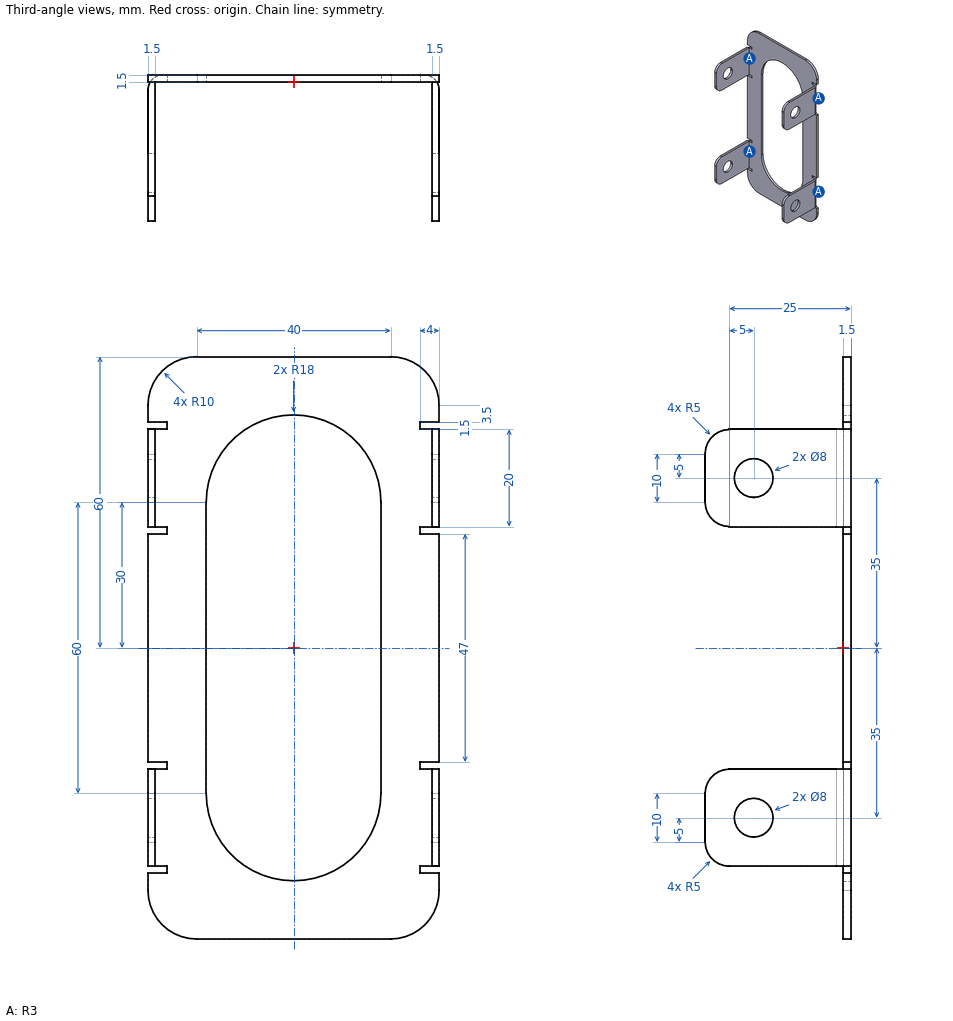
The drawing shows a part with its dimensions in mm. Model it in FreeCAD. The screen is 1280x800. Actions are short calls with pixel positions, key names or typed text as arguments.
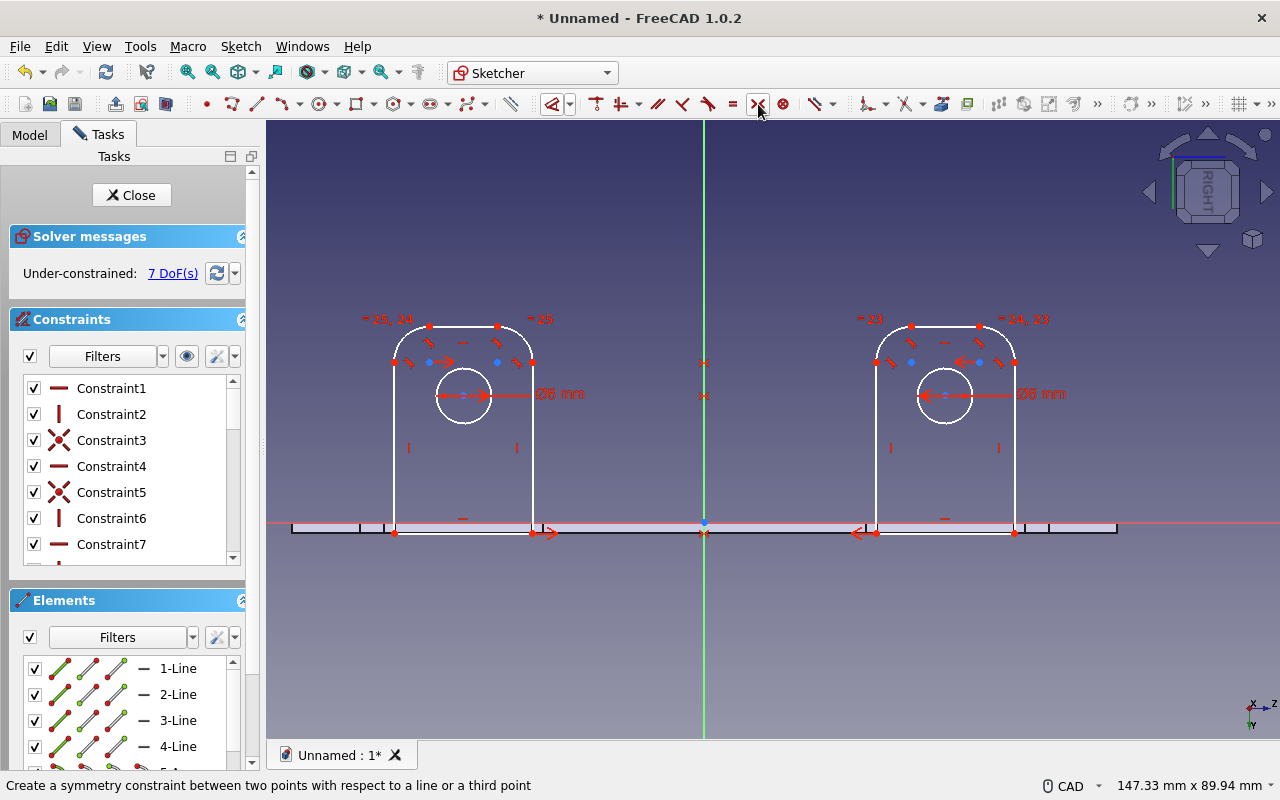
click(896, 331)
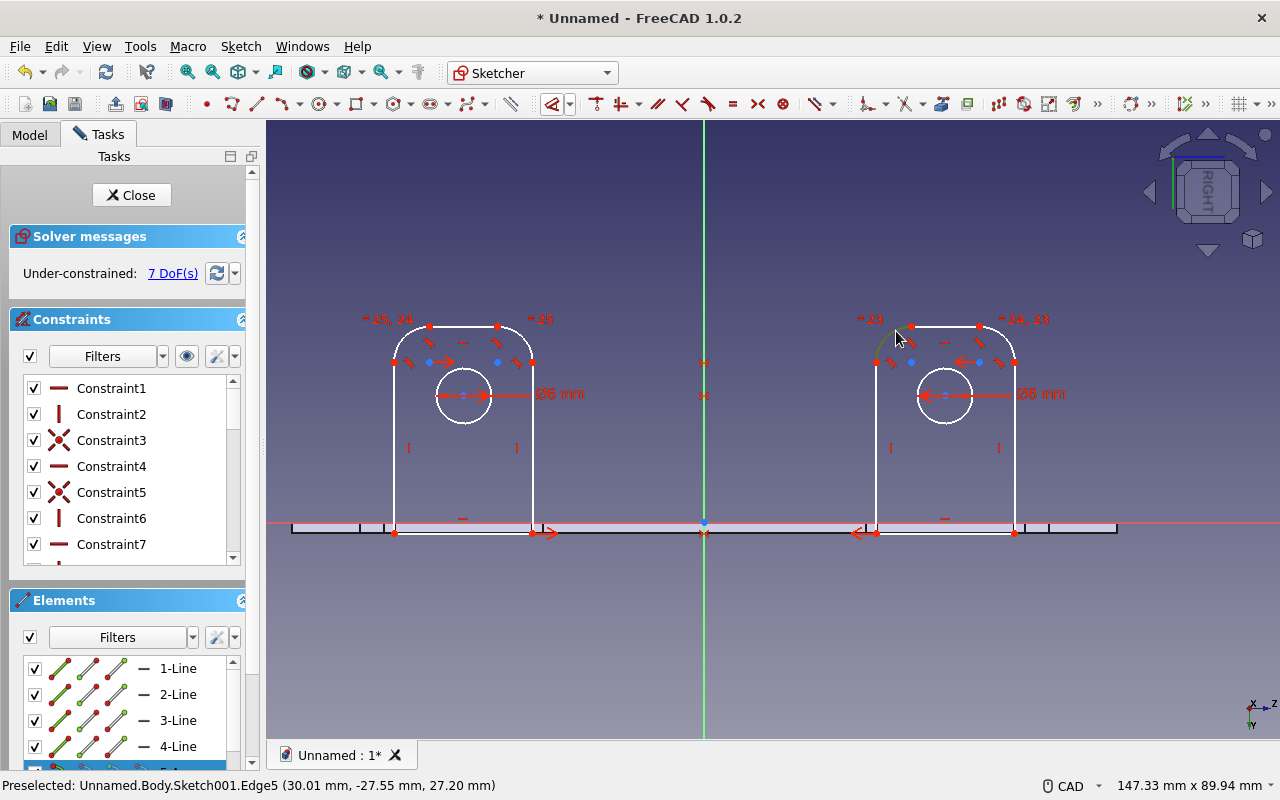
key(k)
key(r)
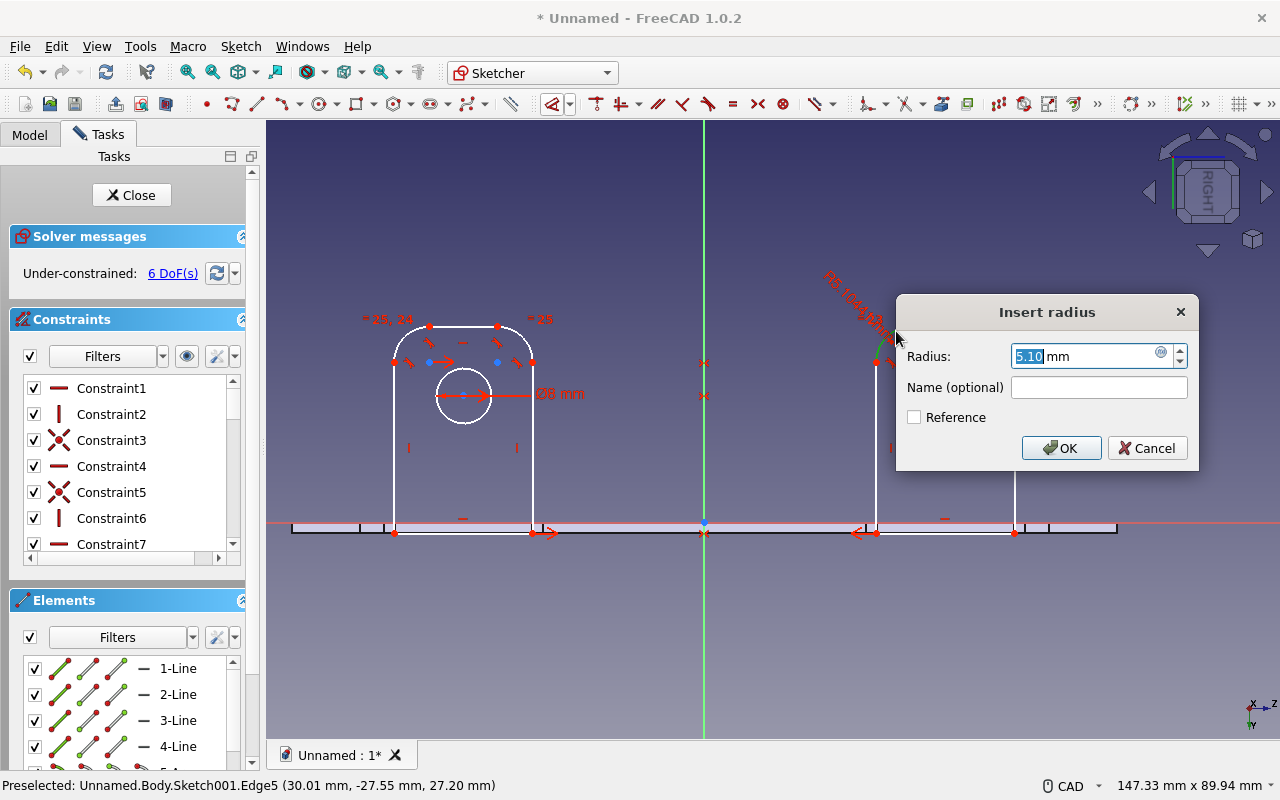
text(5)
key(Return)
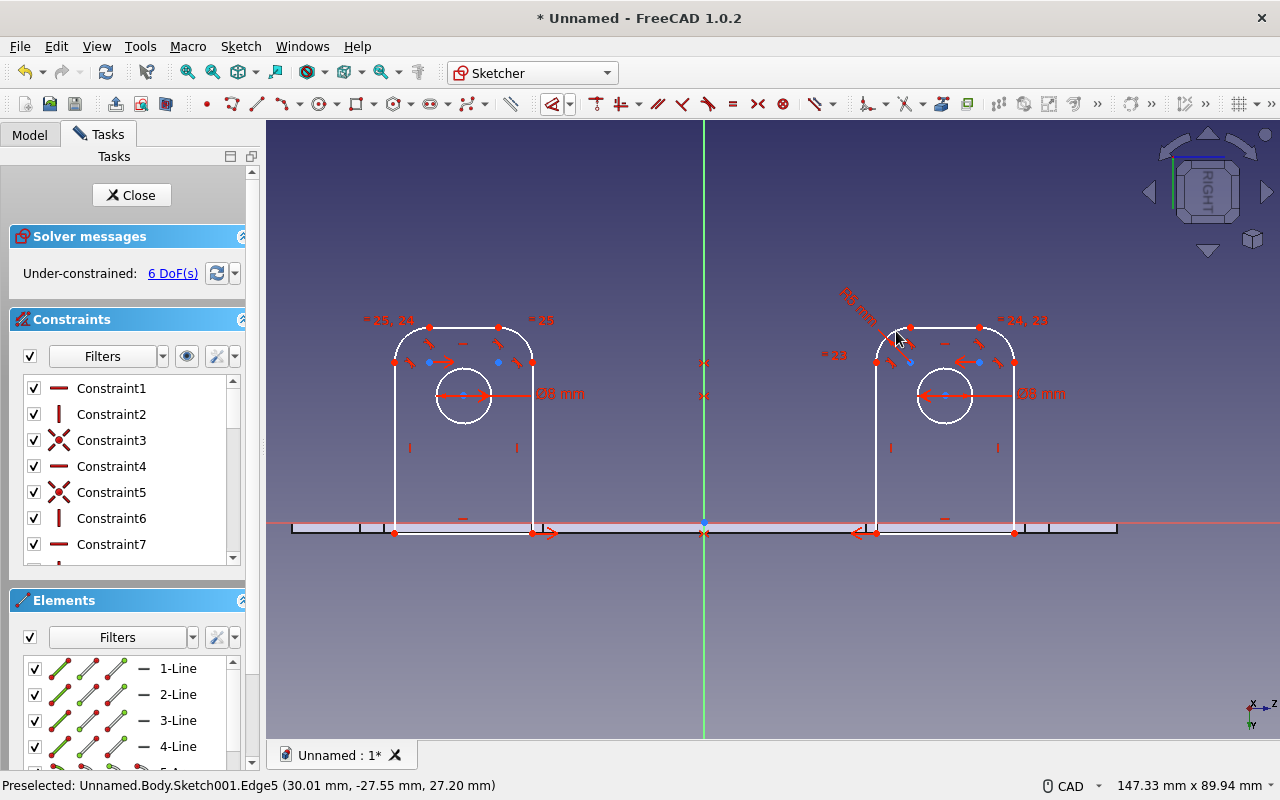
click(959, 328)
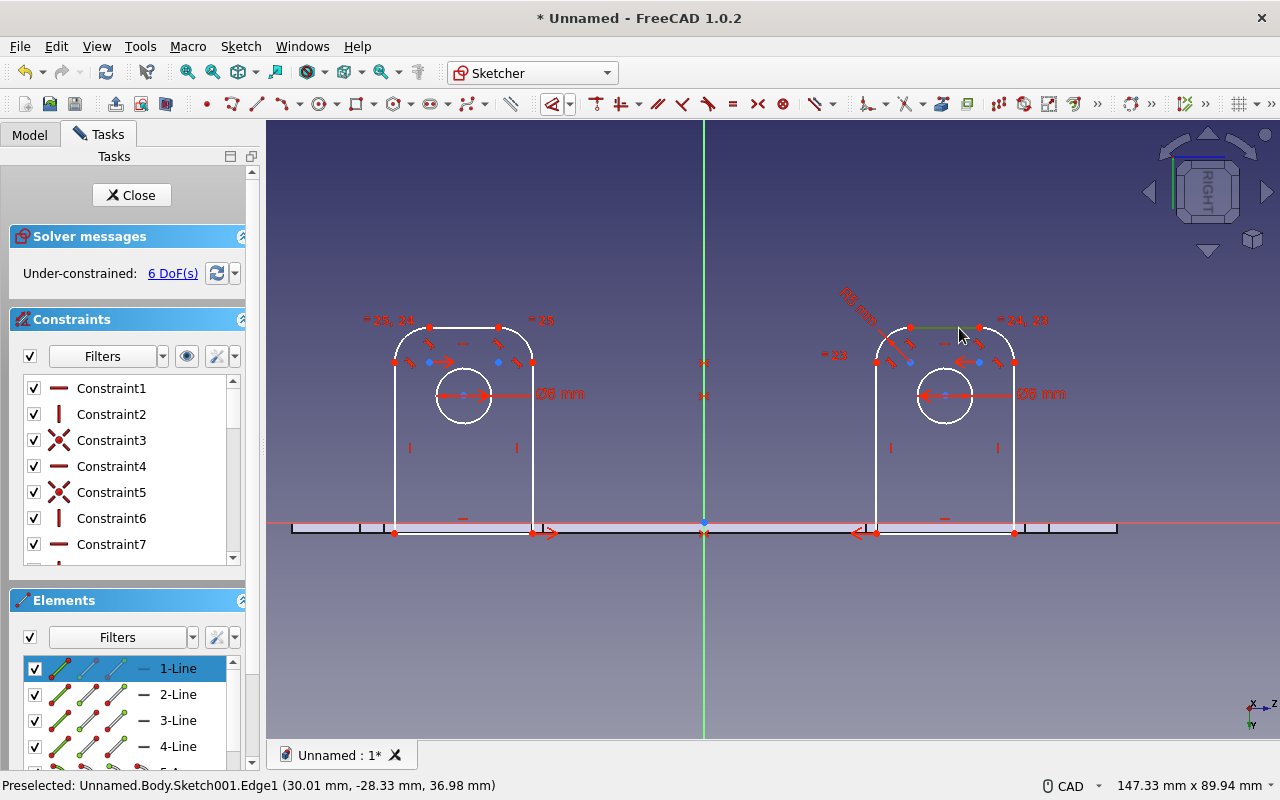
click(570, 104)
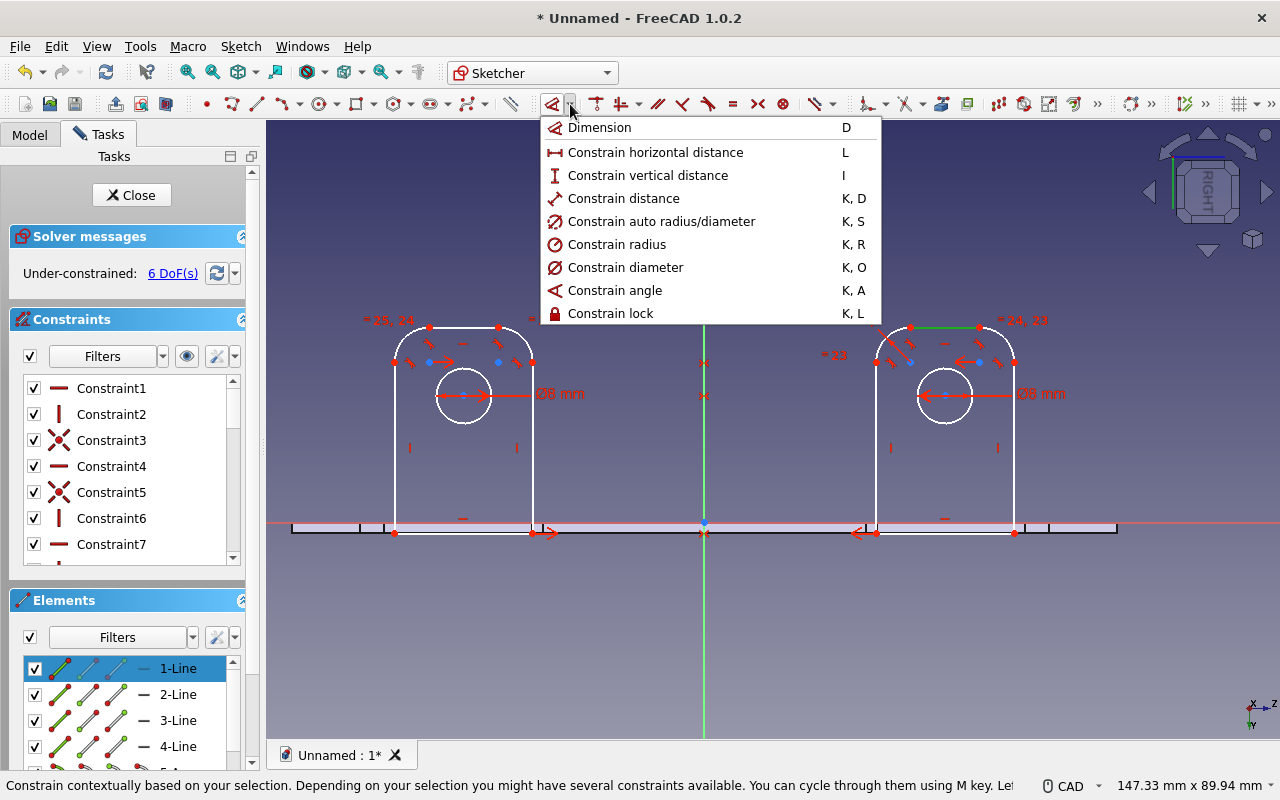
click(711, 152)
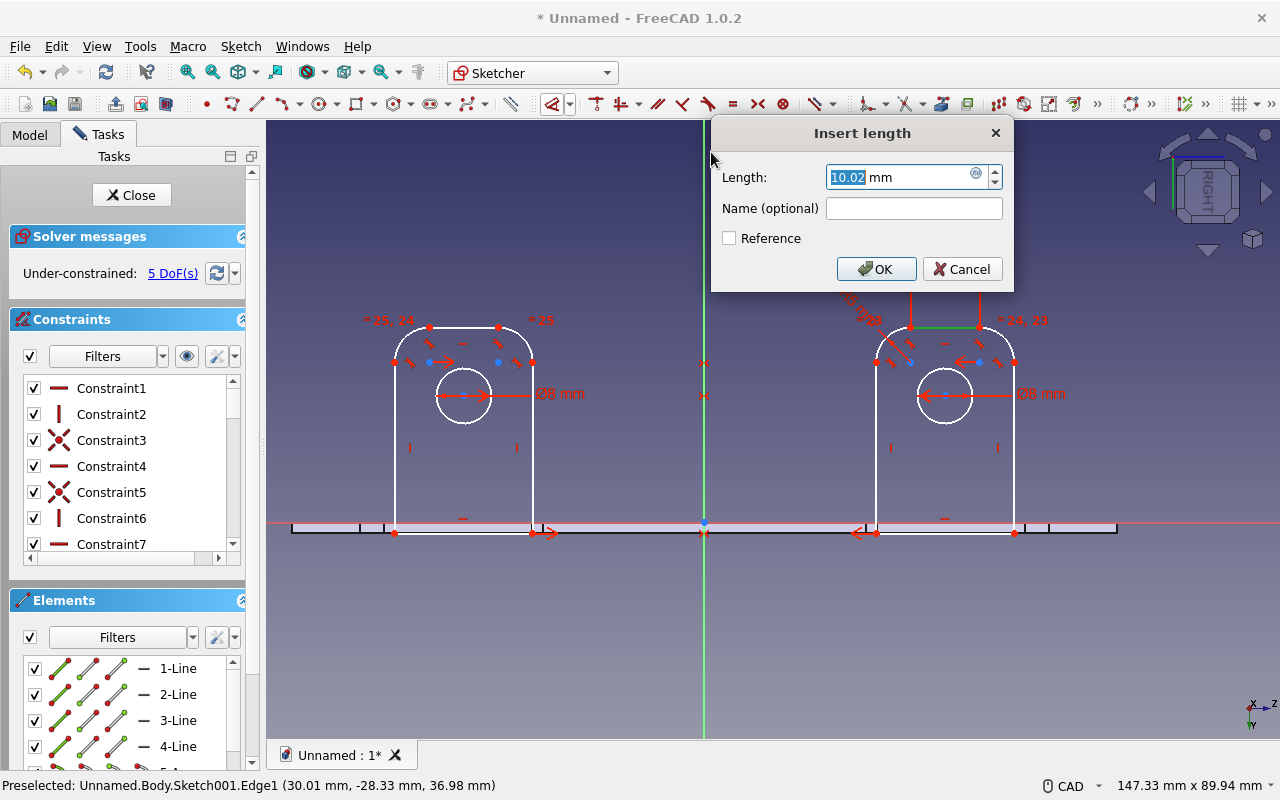
text(10)
key(Return)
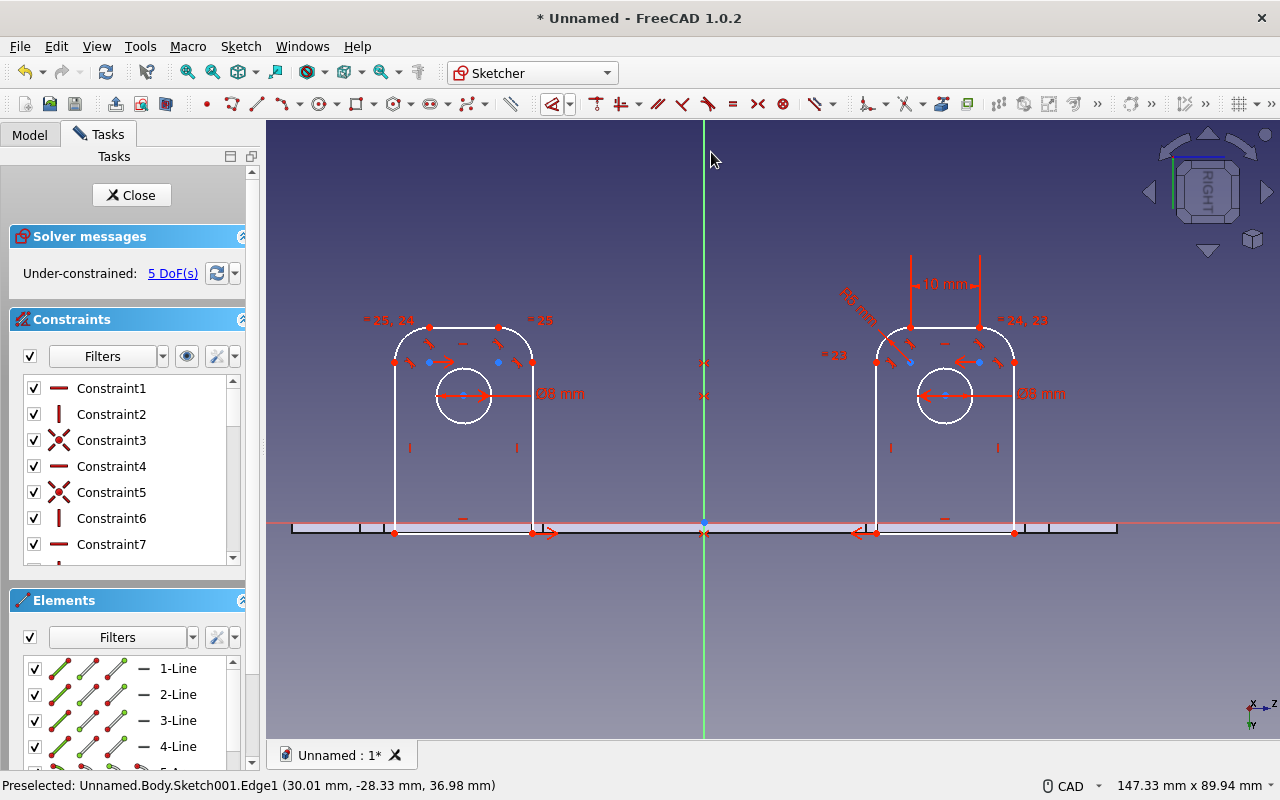
click(876, 413)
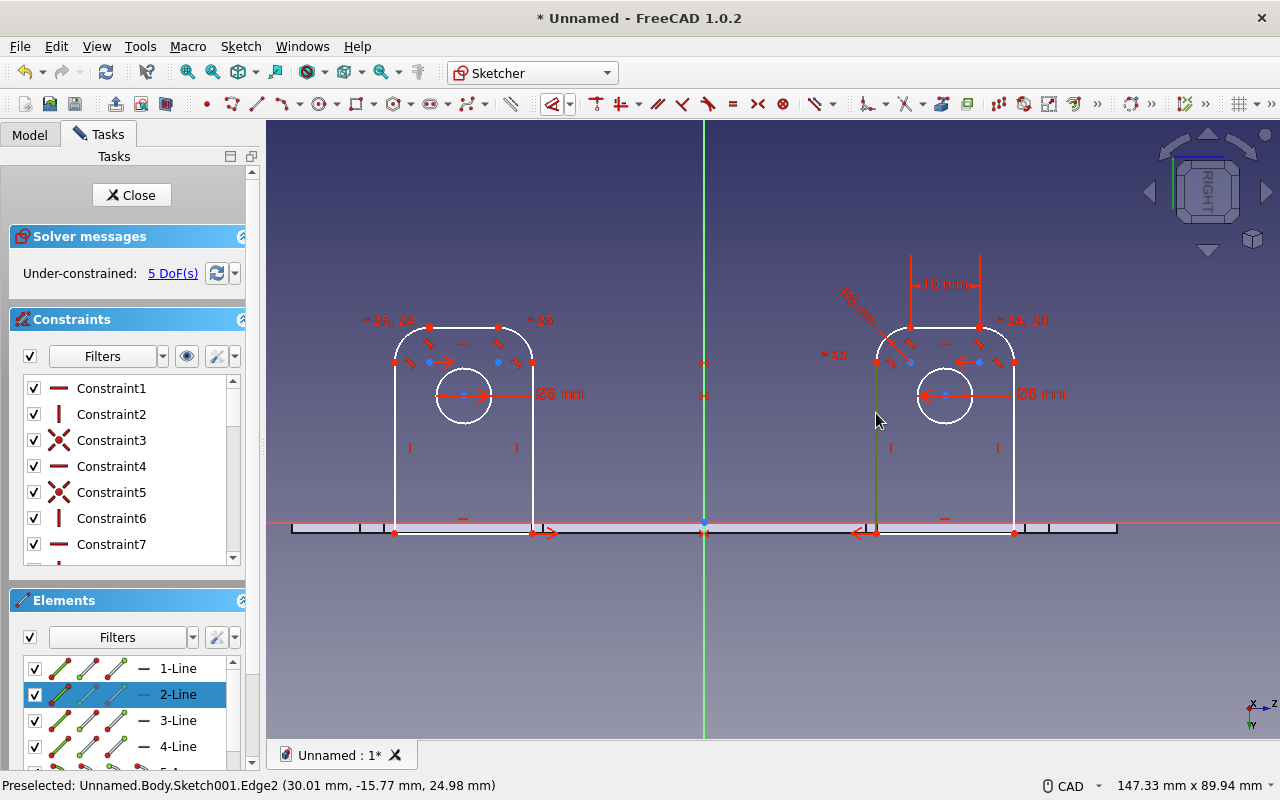
click(570, 104)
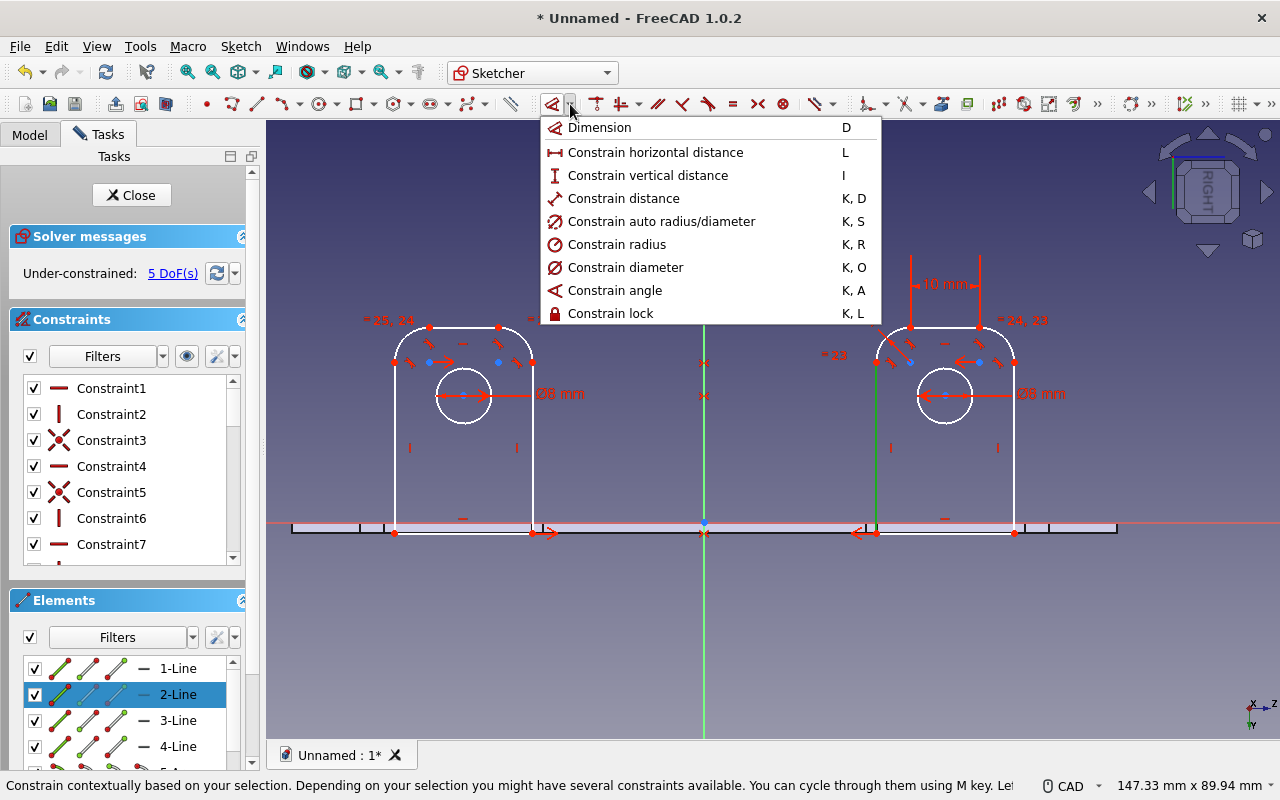
click(711, 176)